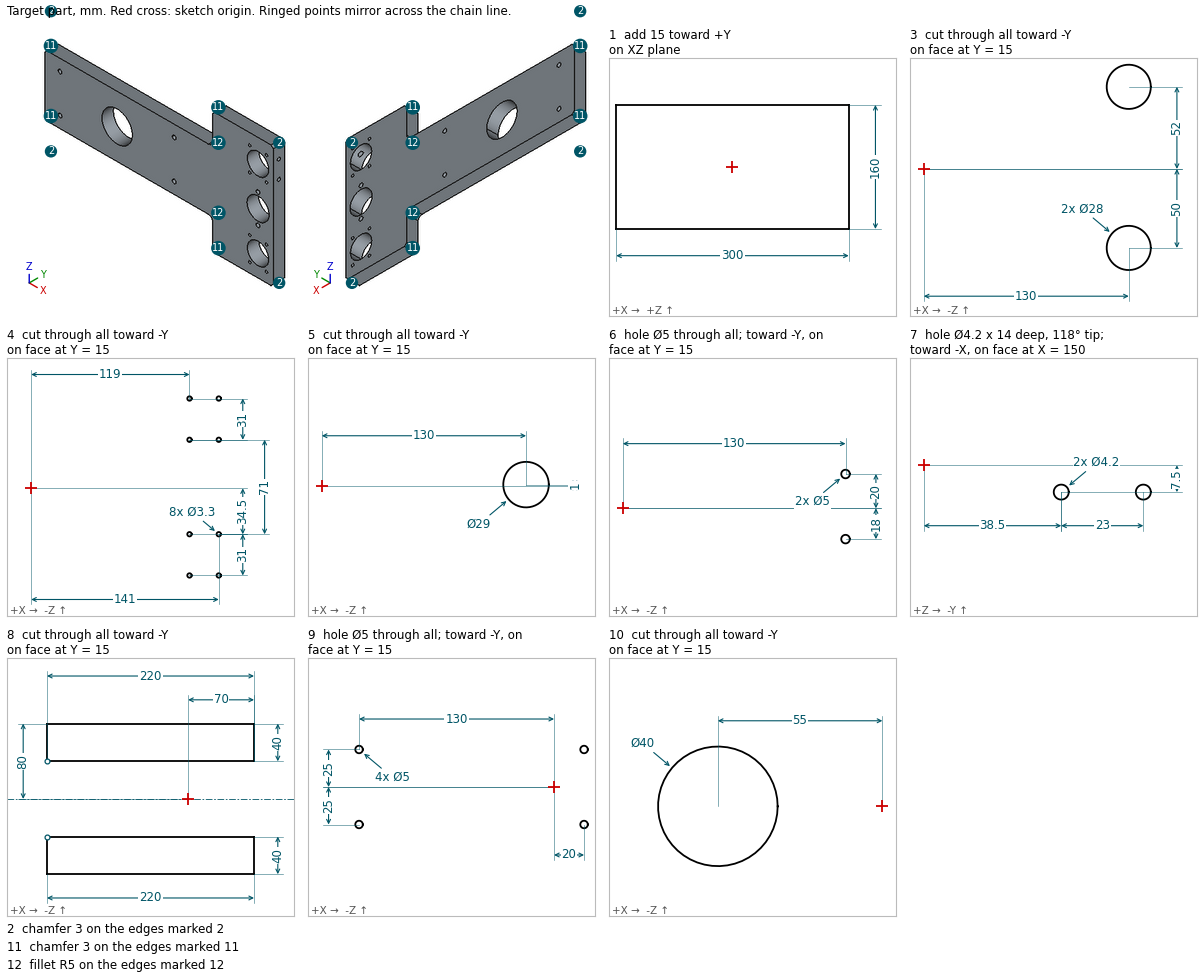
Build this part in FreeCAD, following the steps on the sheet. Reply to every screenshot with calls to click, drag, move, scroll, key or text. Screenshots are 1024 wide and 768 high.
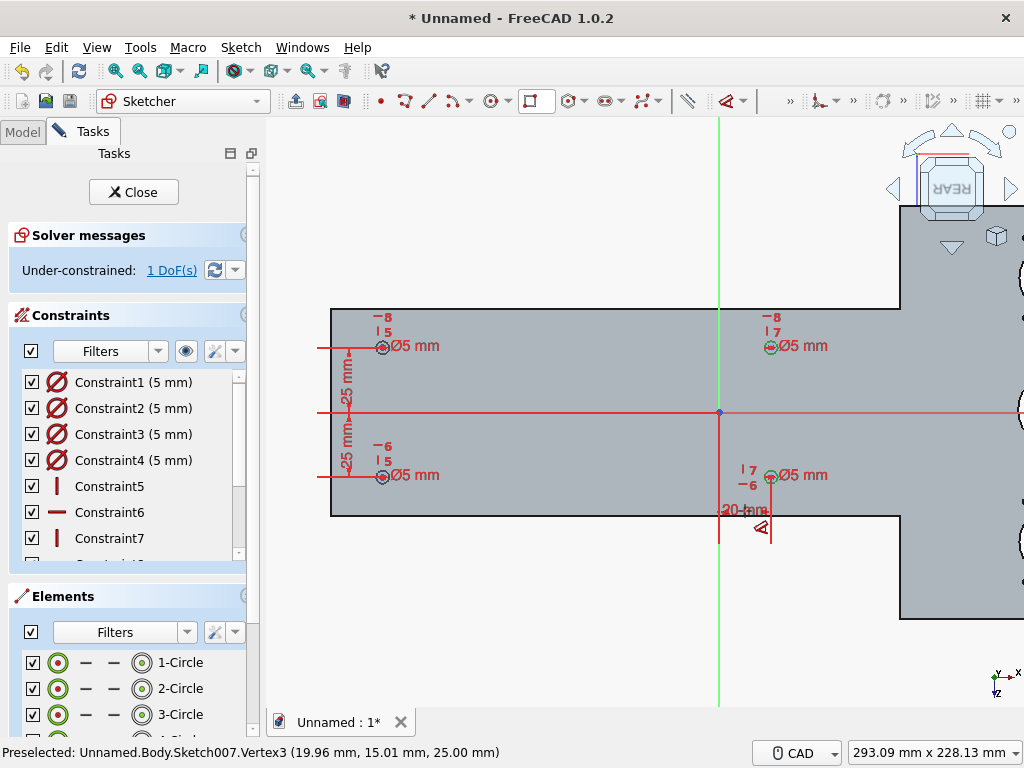
click(383, 348)
click(551, 314)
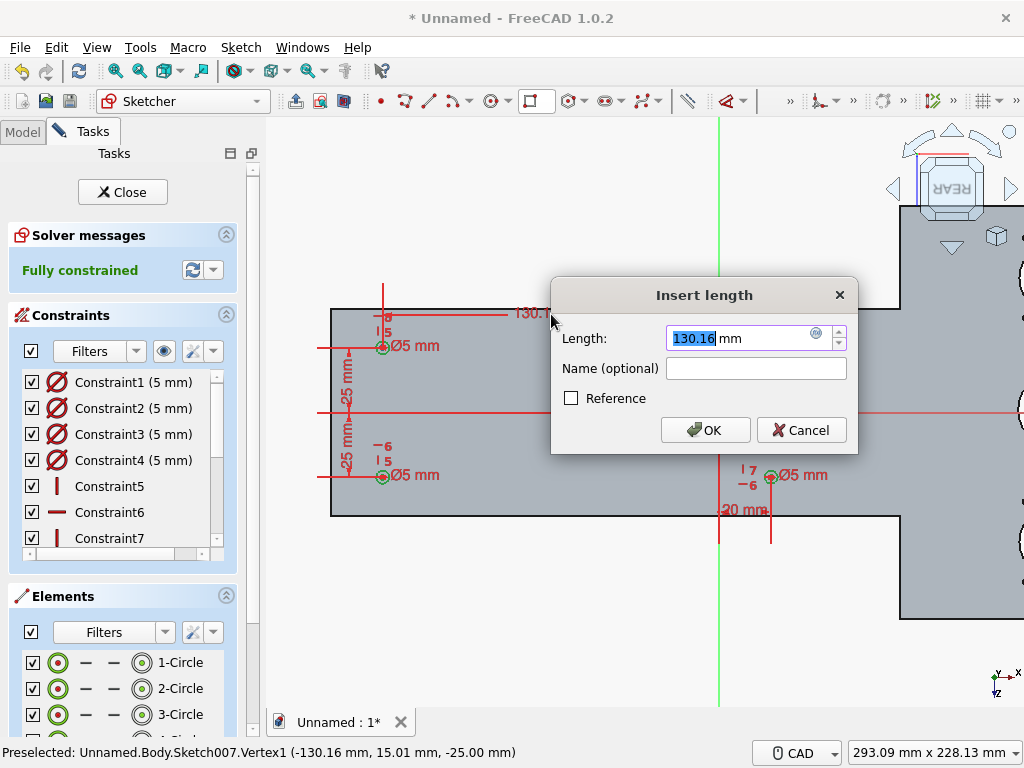
text(130)
key(Return)
key(Escape)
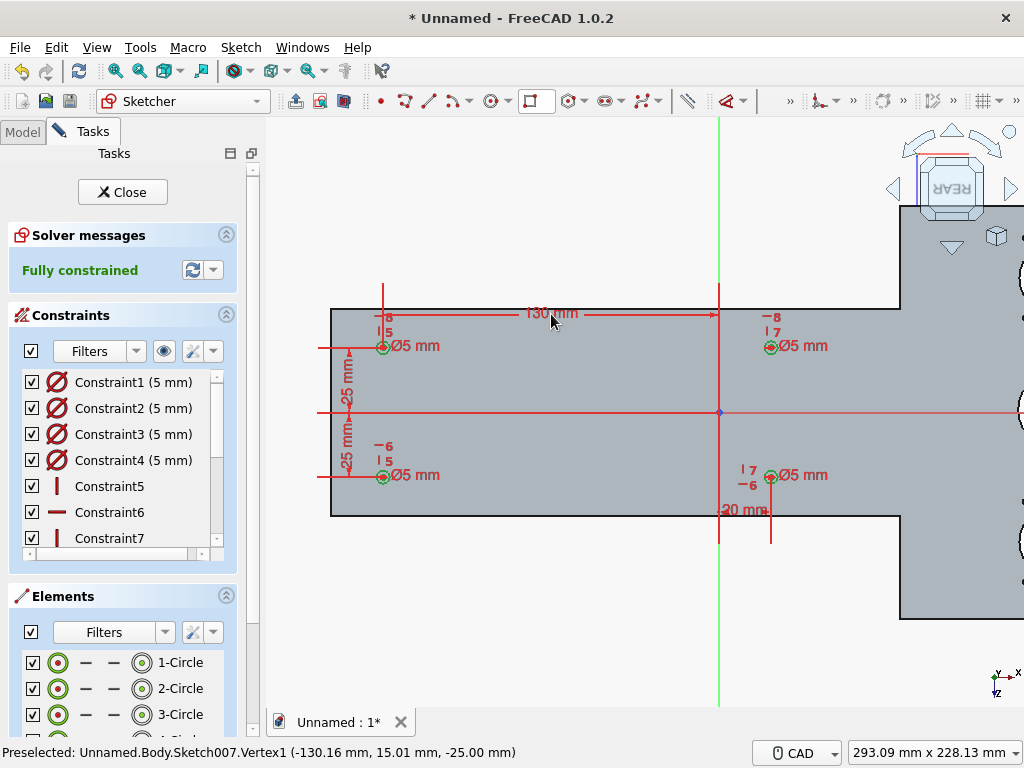
click(123, 192)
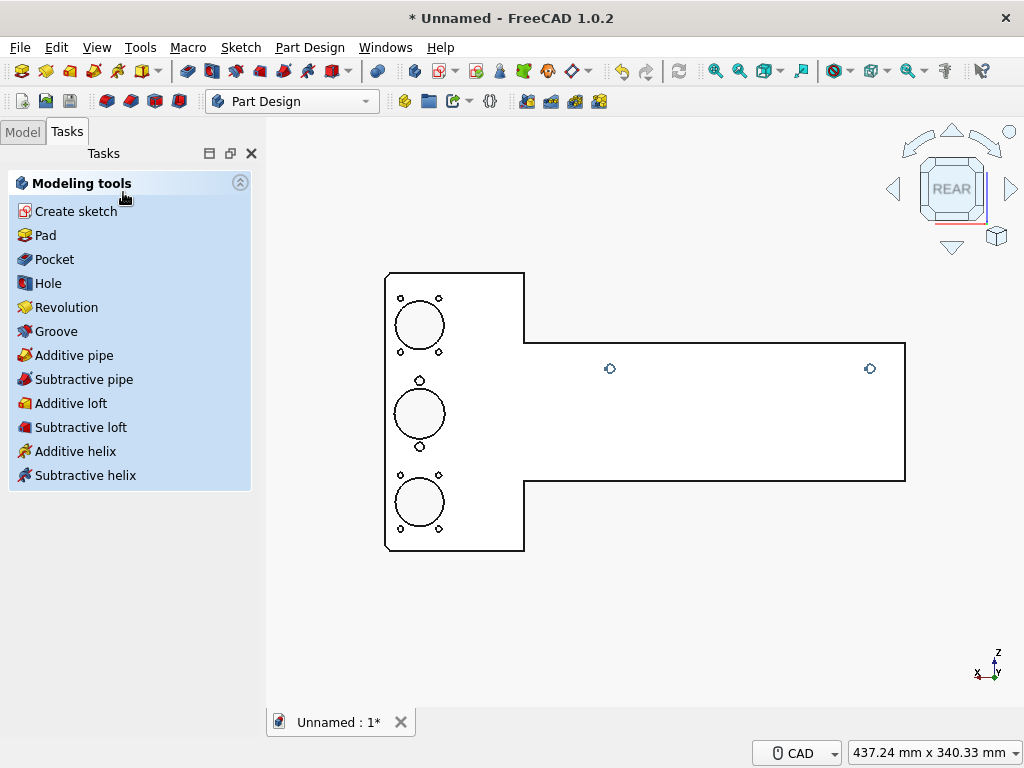
click(212, 72)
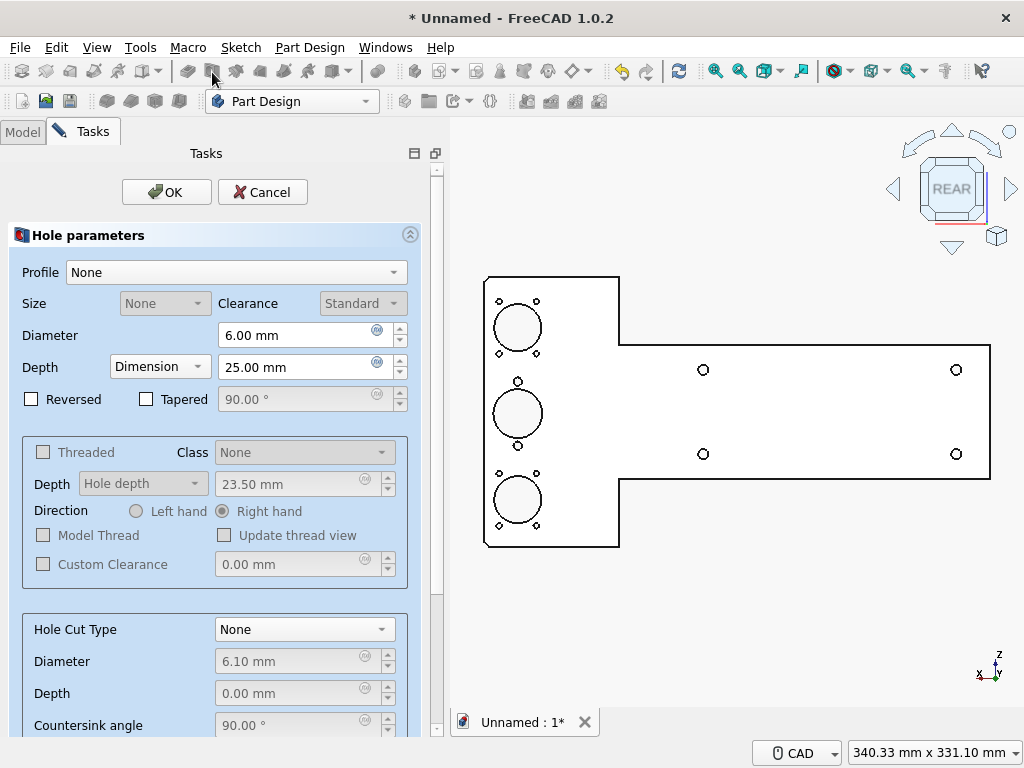
triple_click(305, 335)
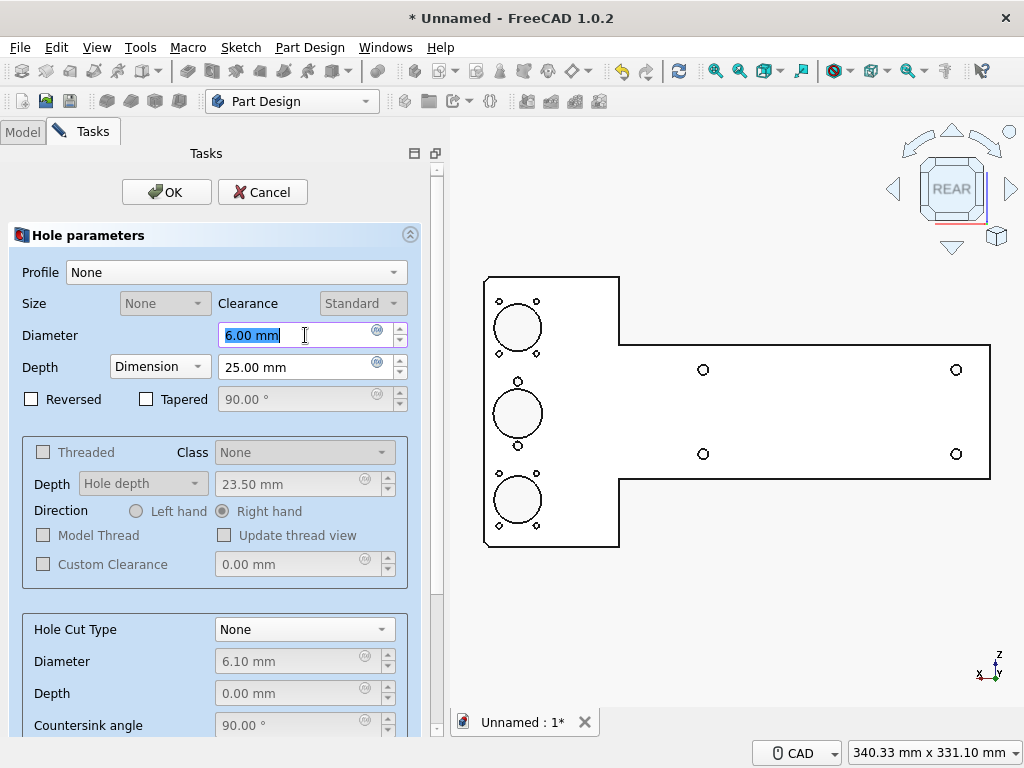
text(5)
key(Tab)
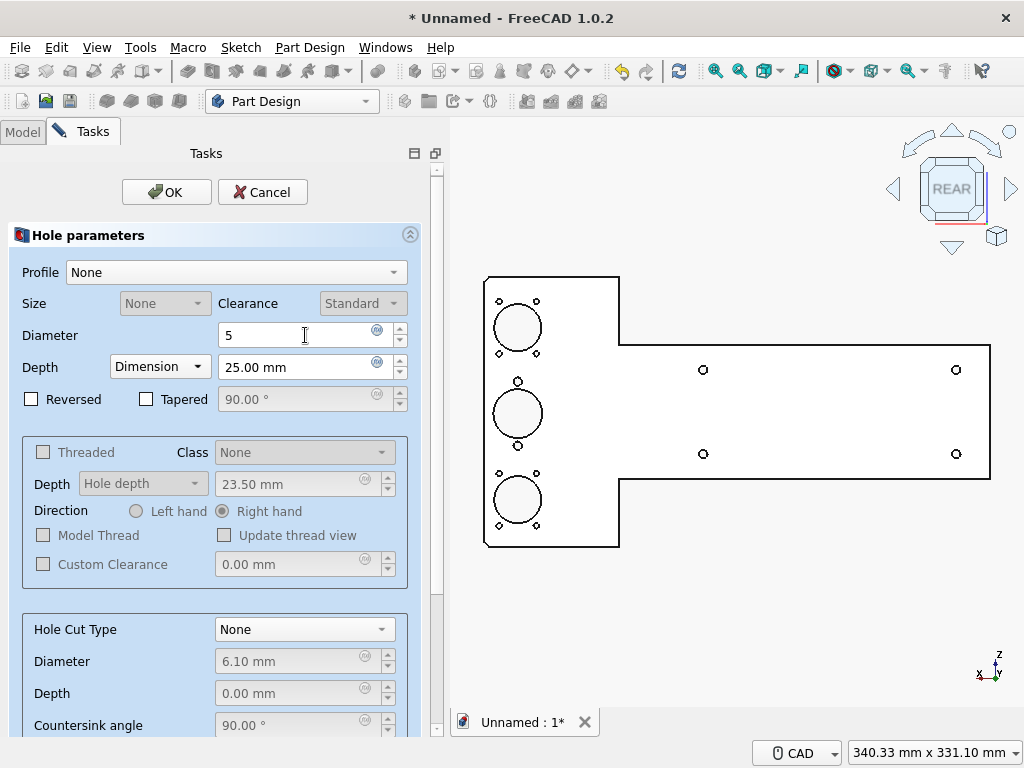
click(161, 366)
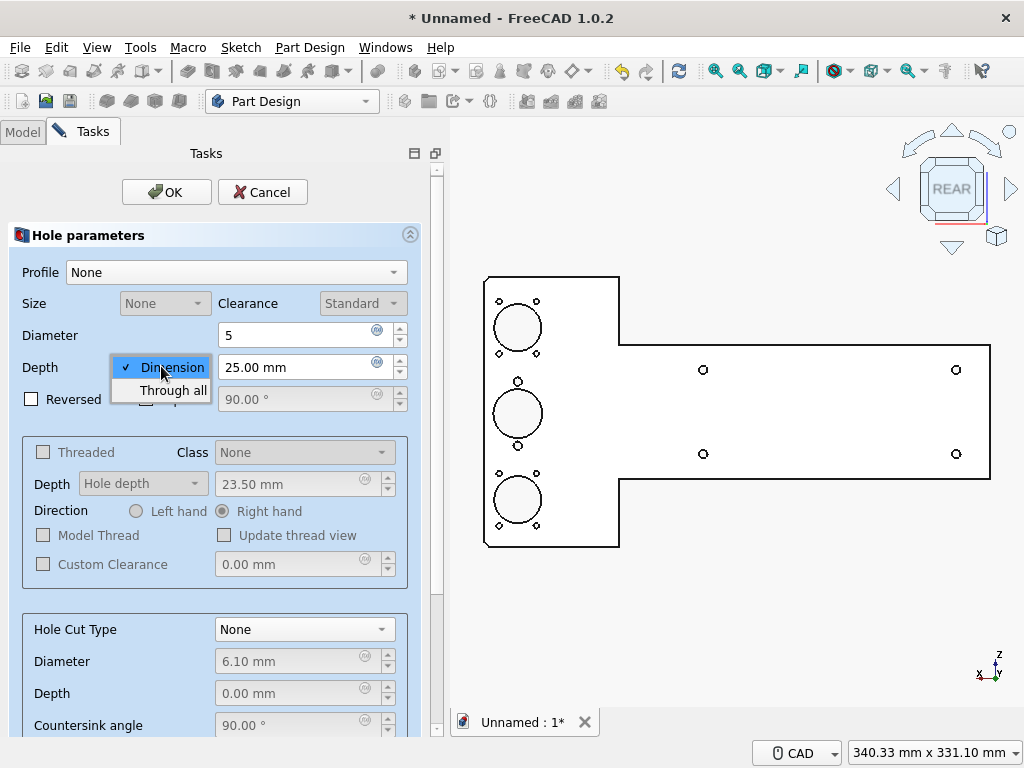
click(160, 390)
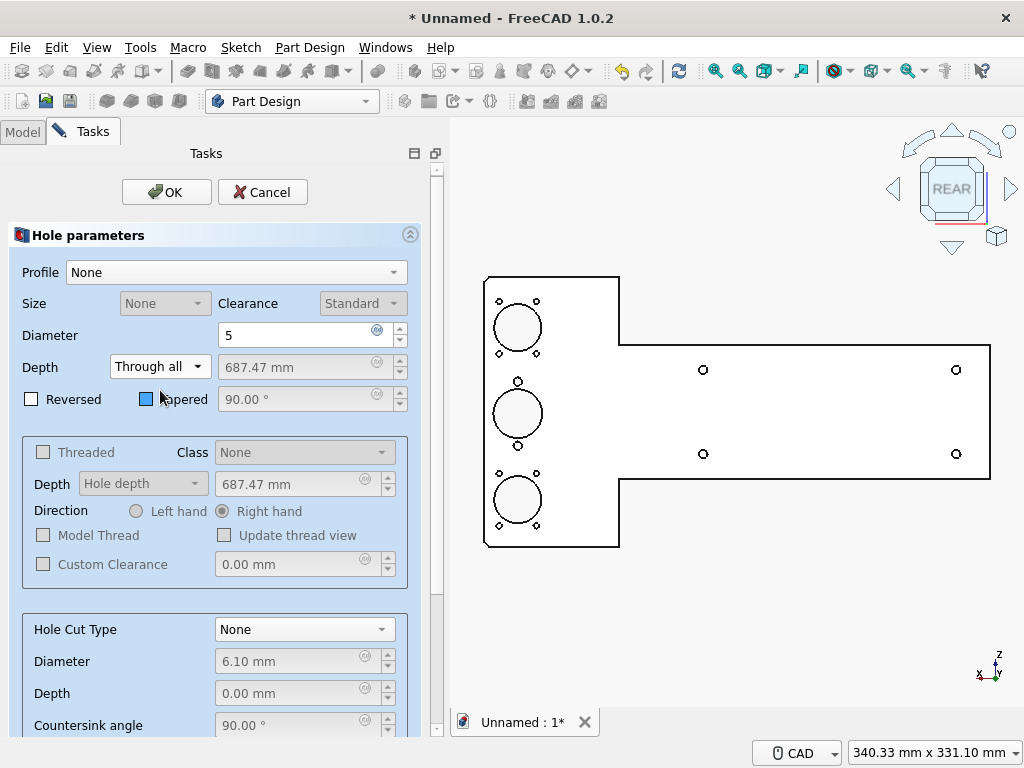
click(167, 192)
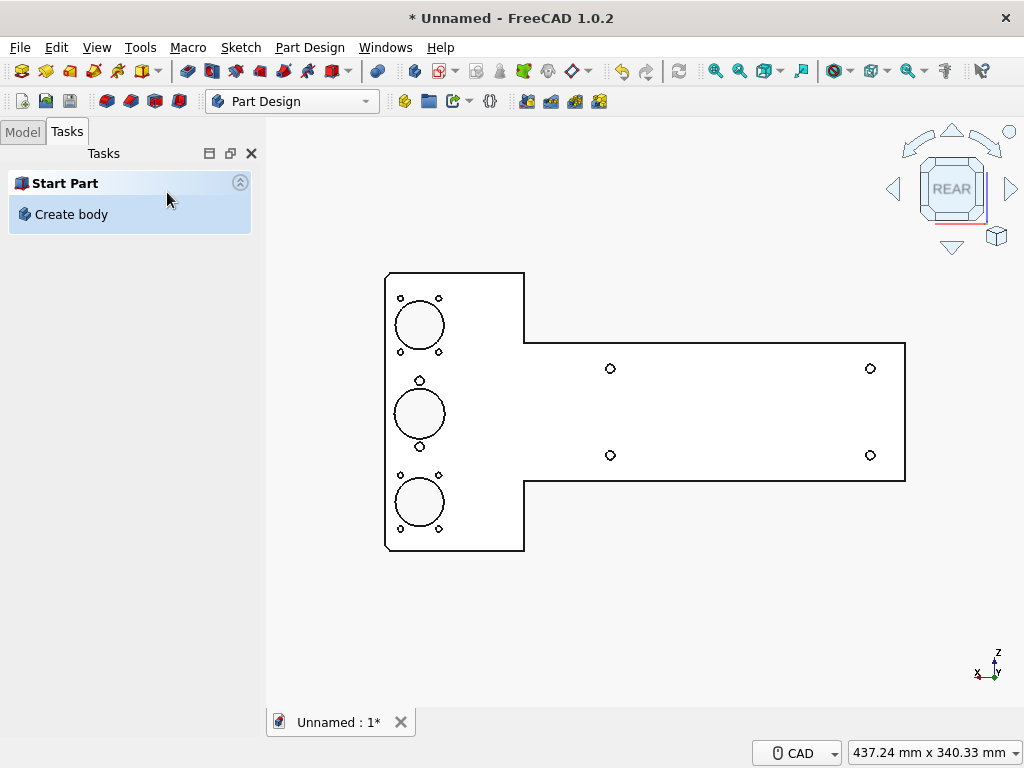
click(719, 411)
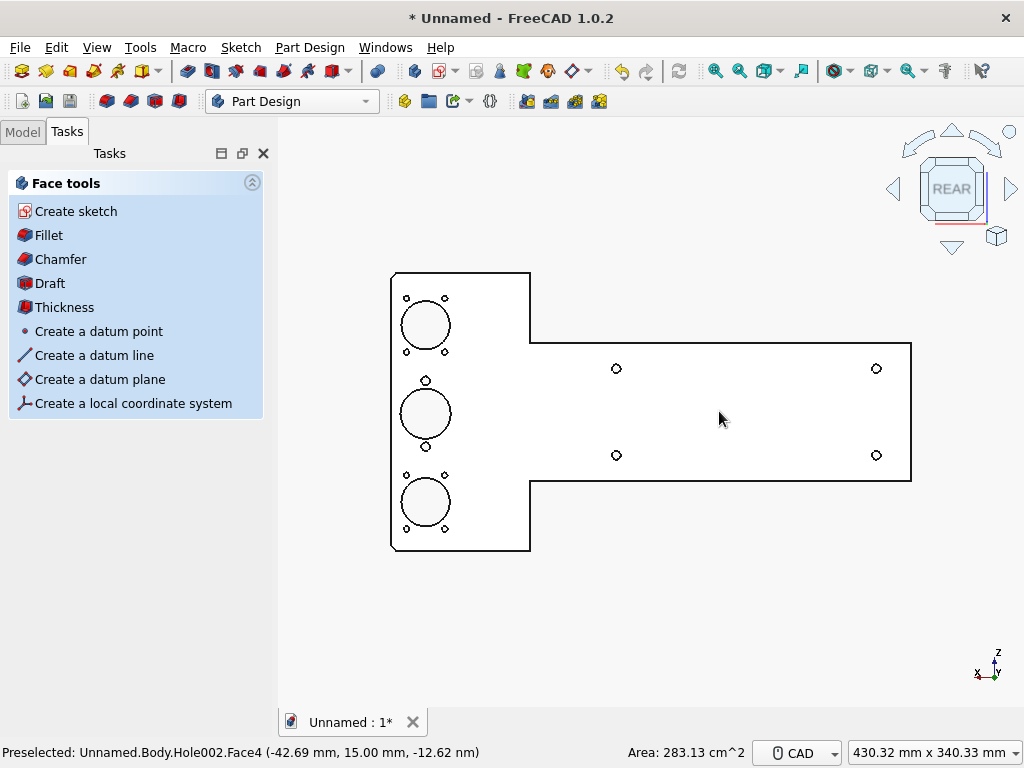
click(440, 72)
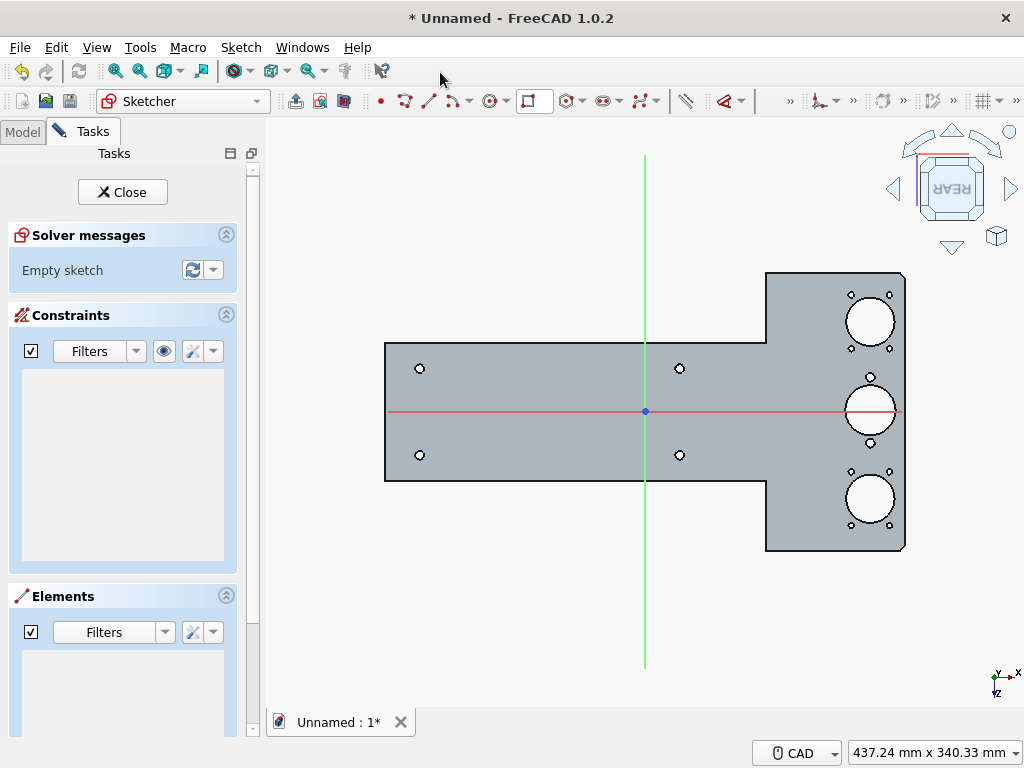
scroll(581, 412, up, 6)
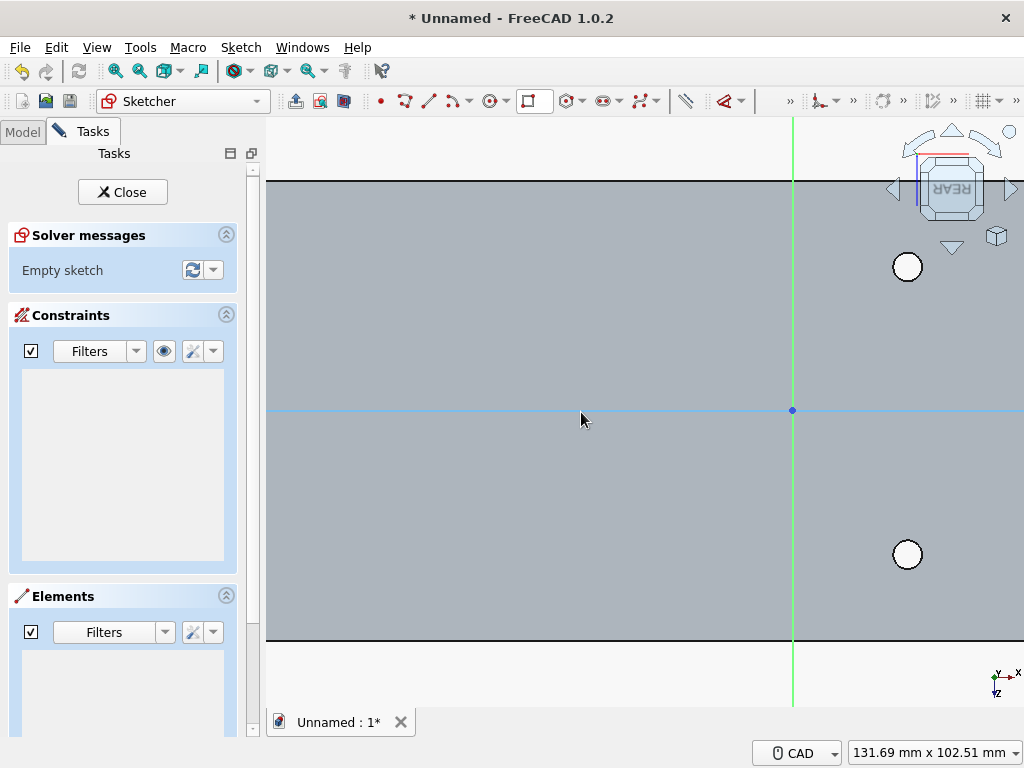
click(490, 102)